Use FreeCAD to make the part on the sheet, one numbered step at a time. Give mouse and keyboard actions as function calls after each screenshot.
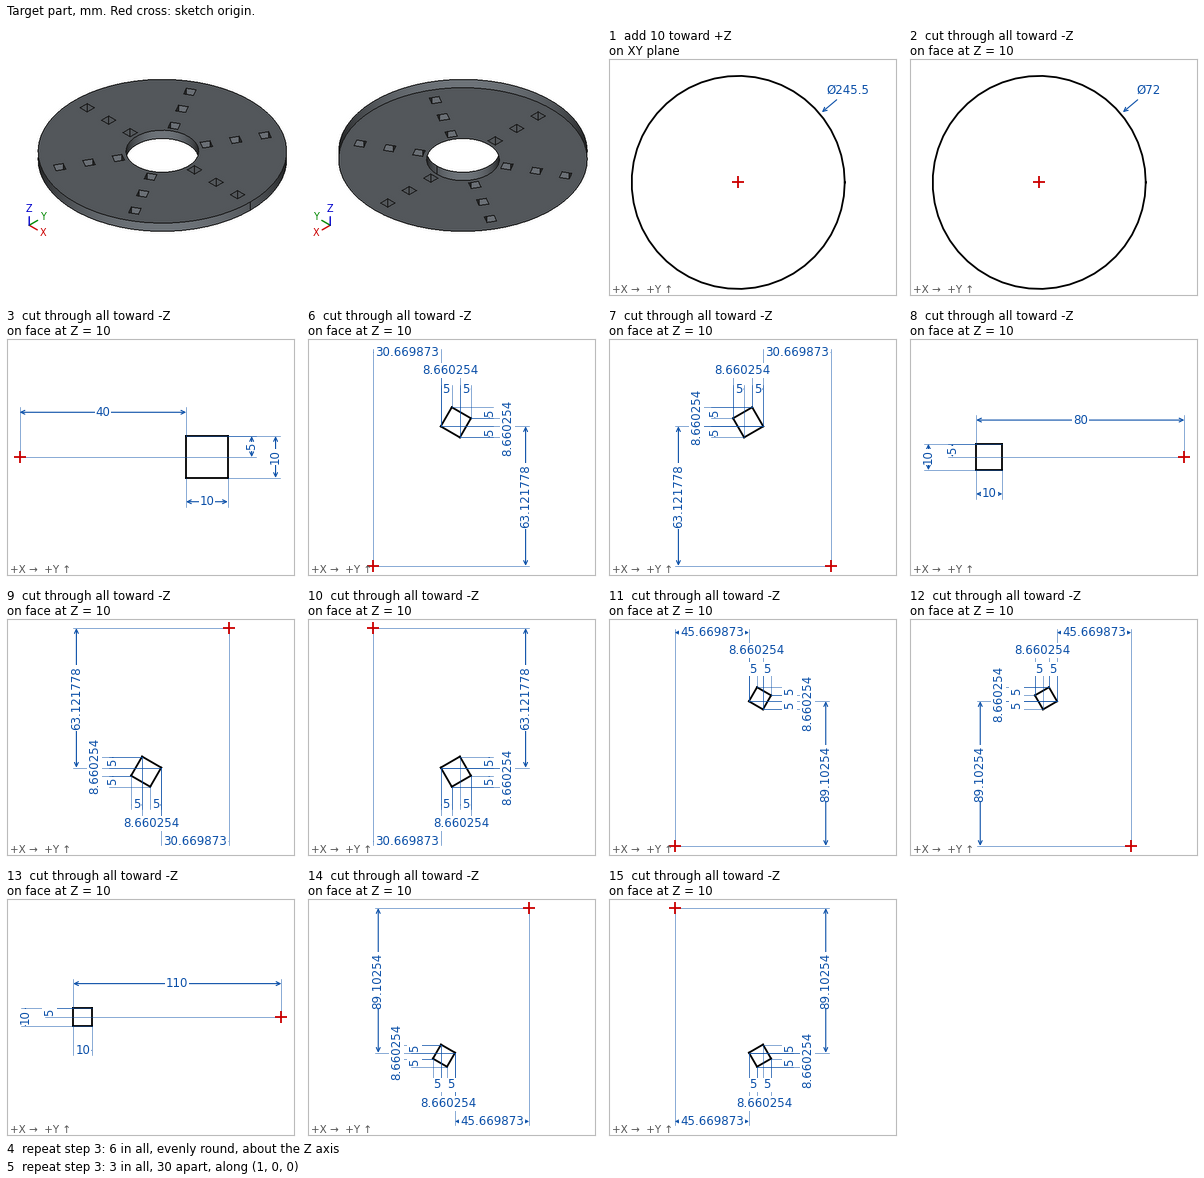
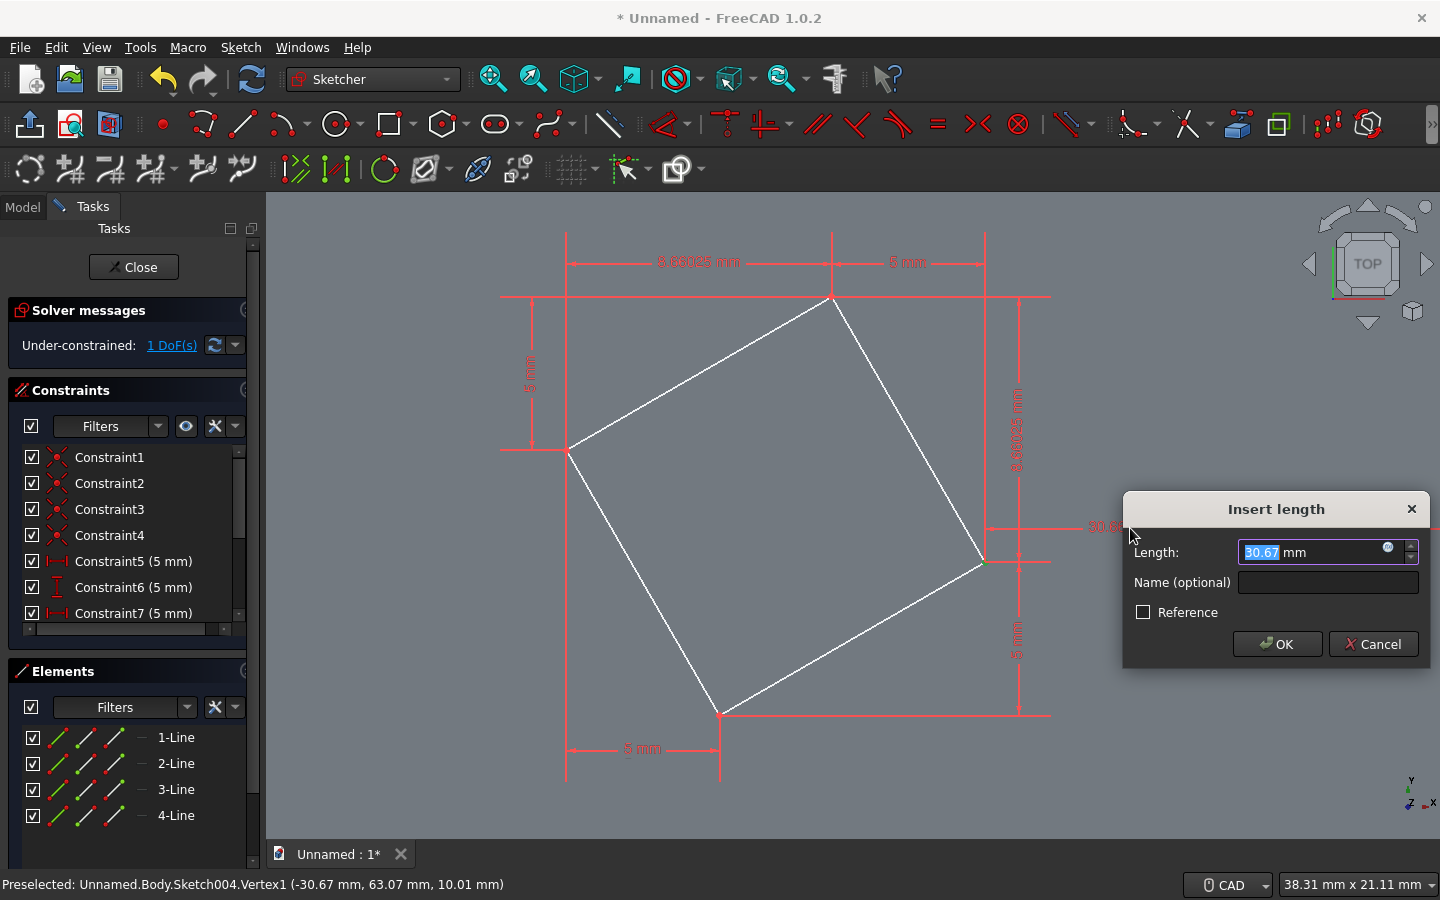
text(30.669873)
key(Return)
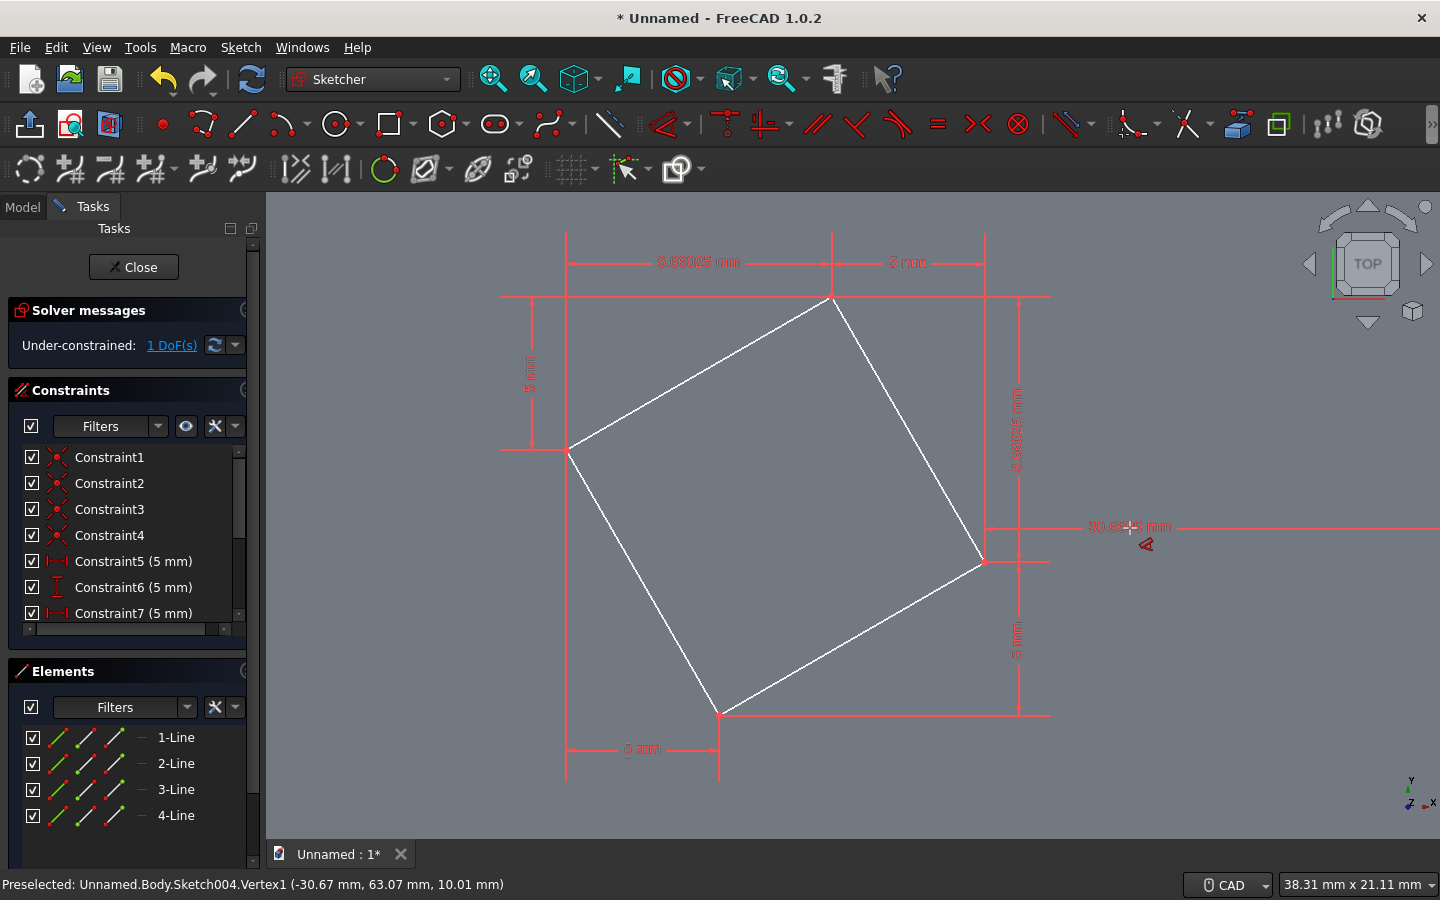
click(985, 562)
click(951, 687)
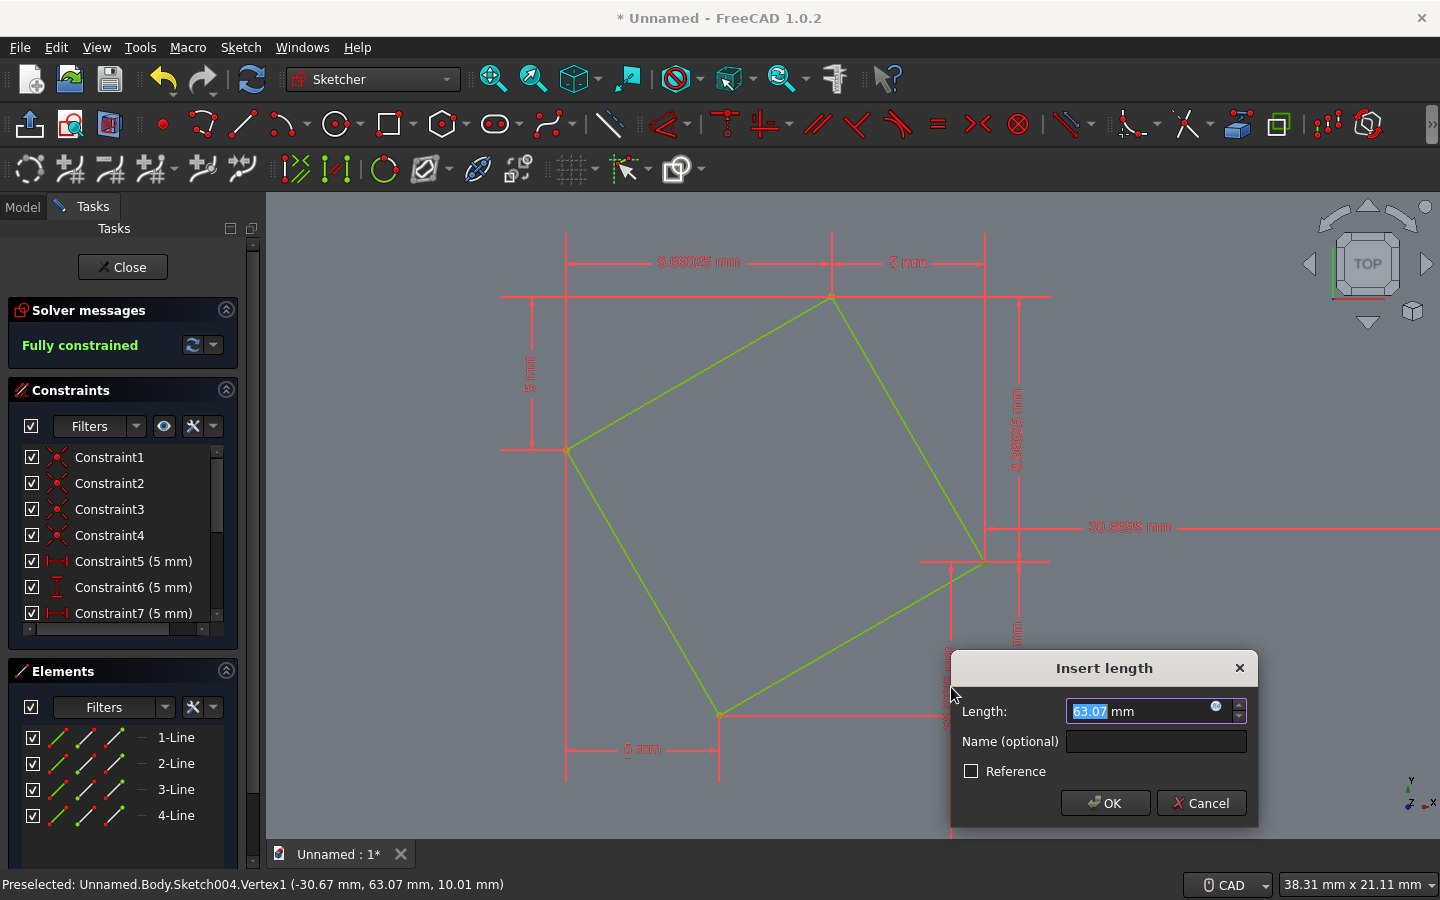
text(63.121778)
key(Return)
key(Escape)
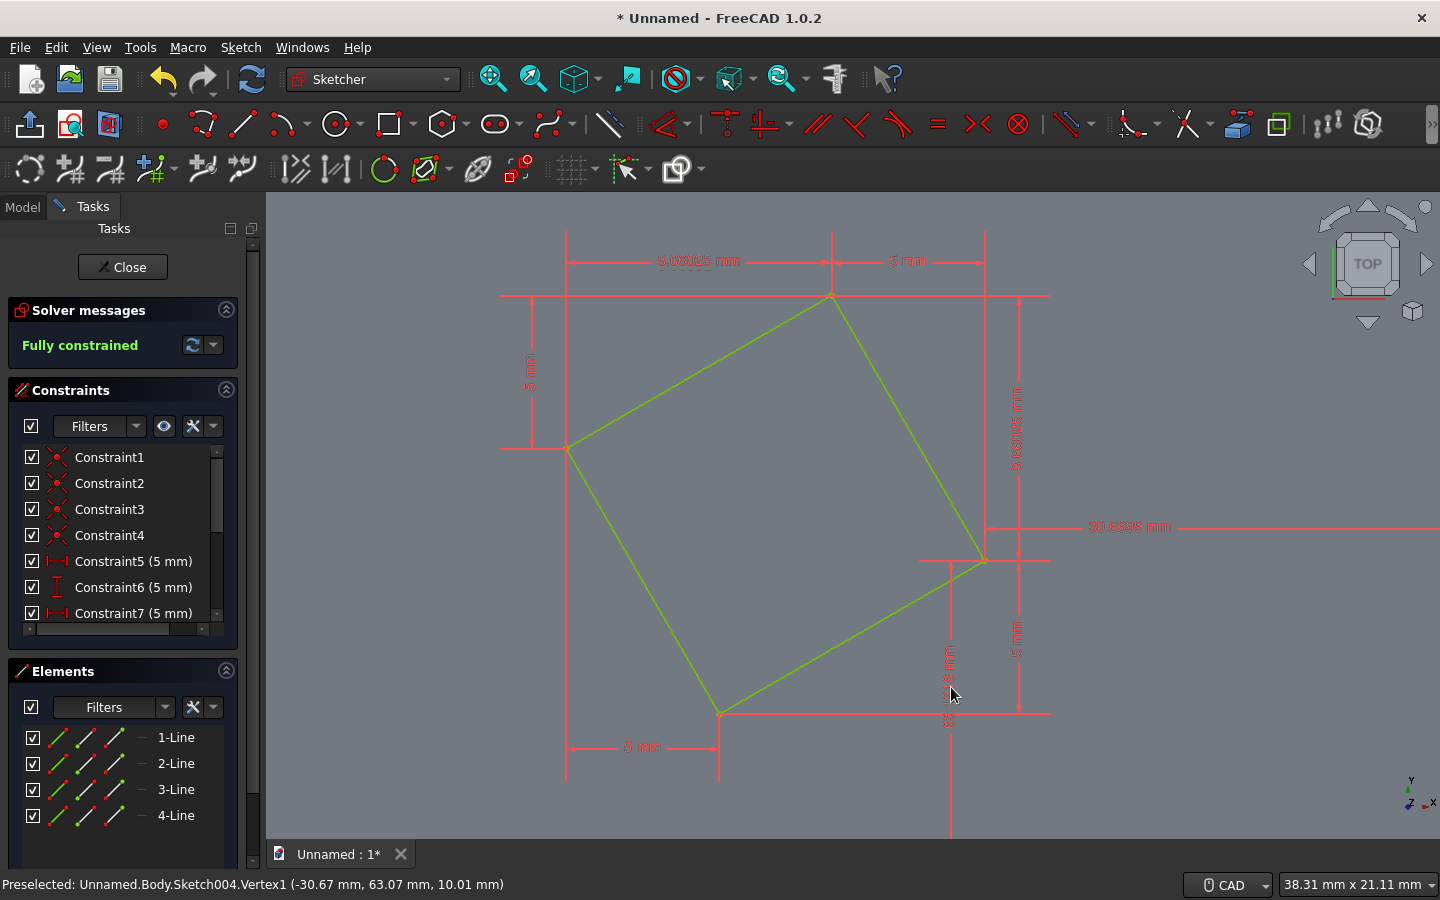
click(123, 267)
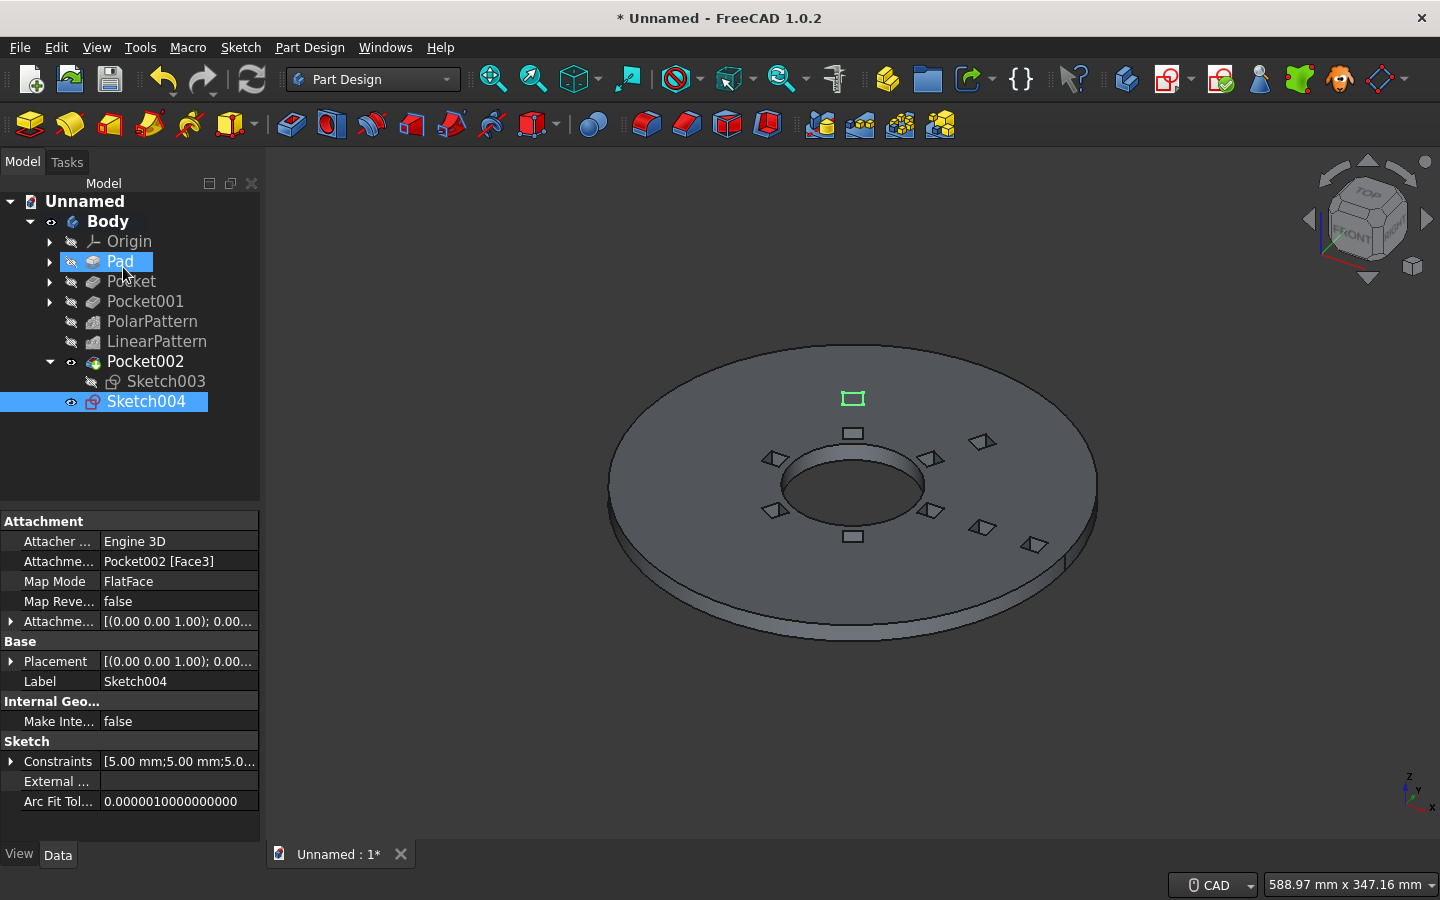
click(292, 124)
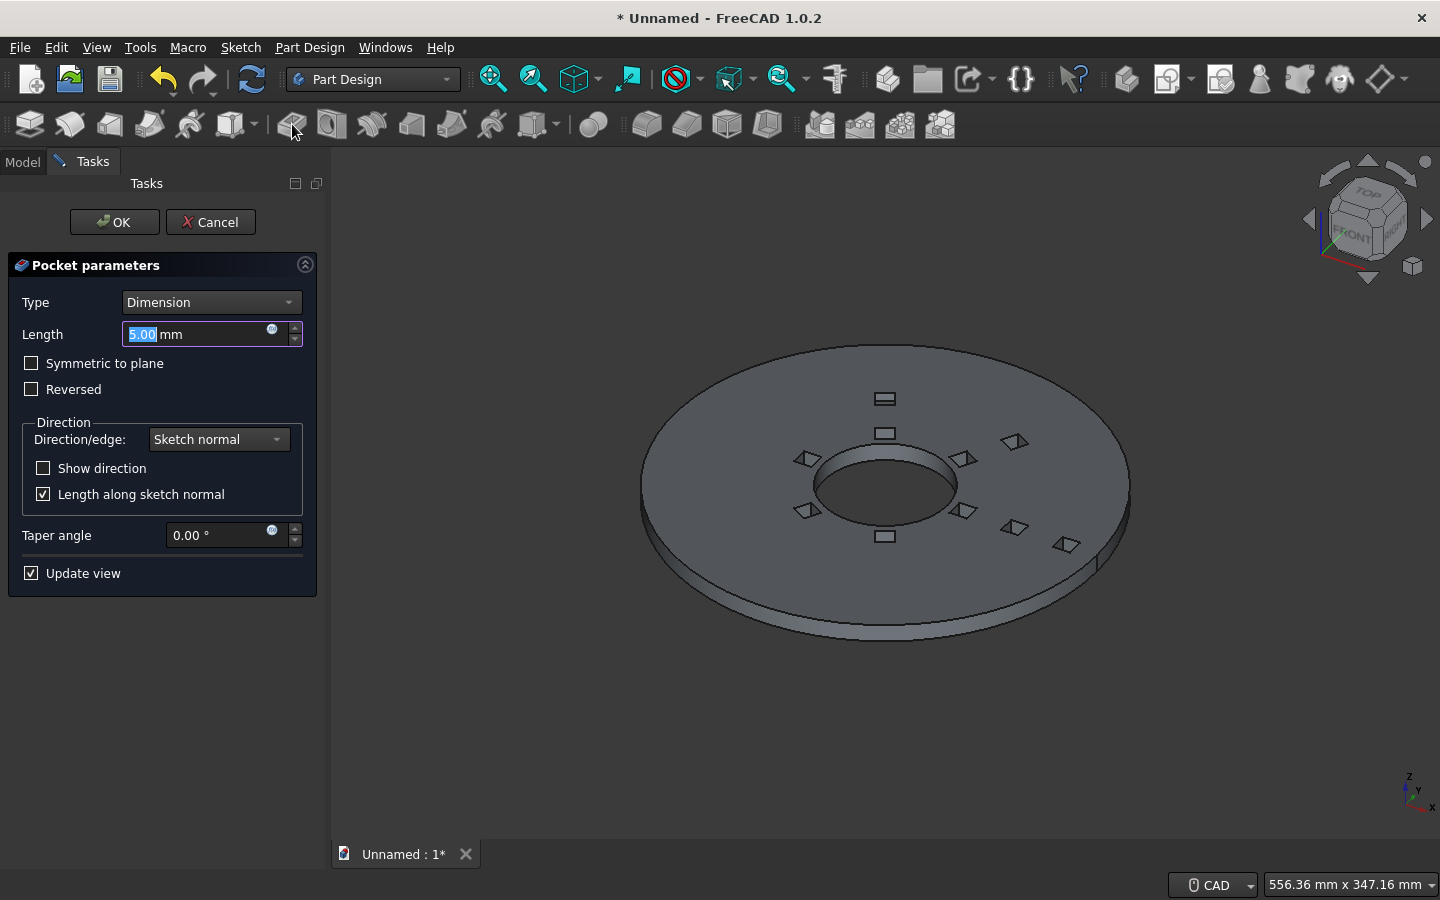
click(212, 302)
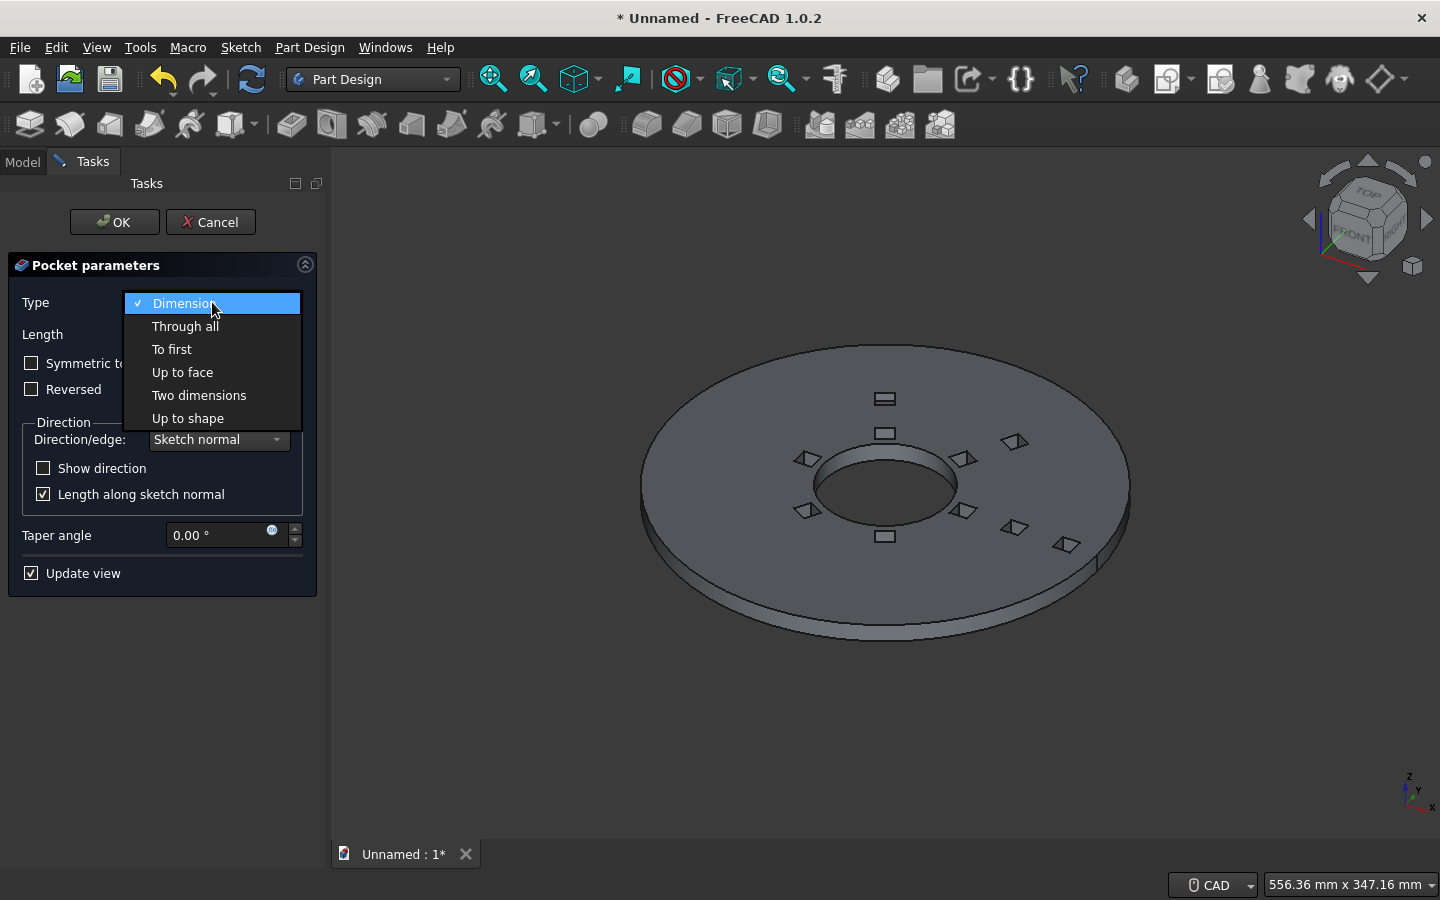
click(212, 326)